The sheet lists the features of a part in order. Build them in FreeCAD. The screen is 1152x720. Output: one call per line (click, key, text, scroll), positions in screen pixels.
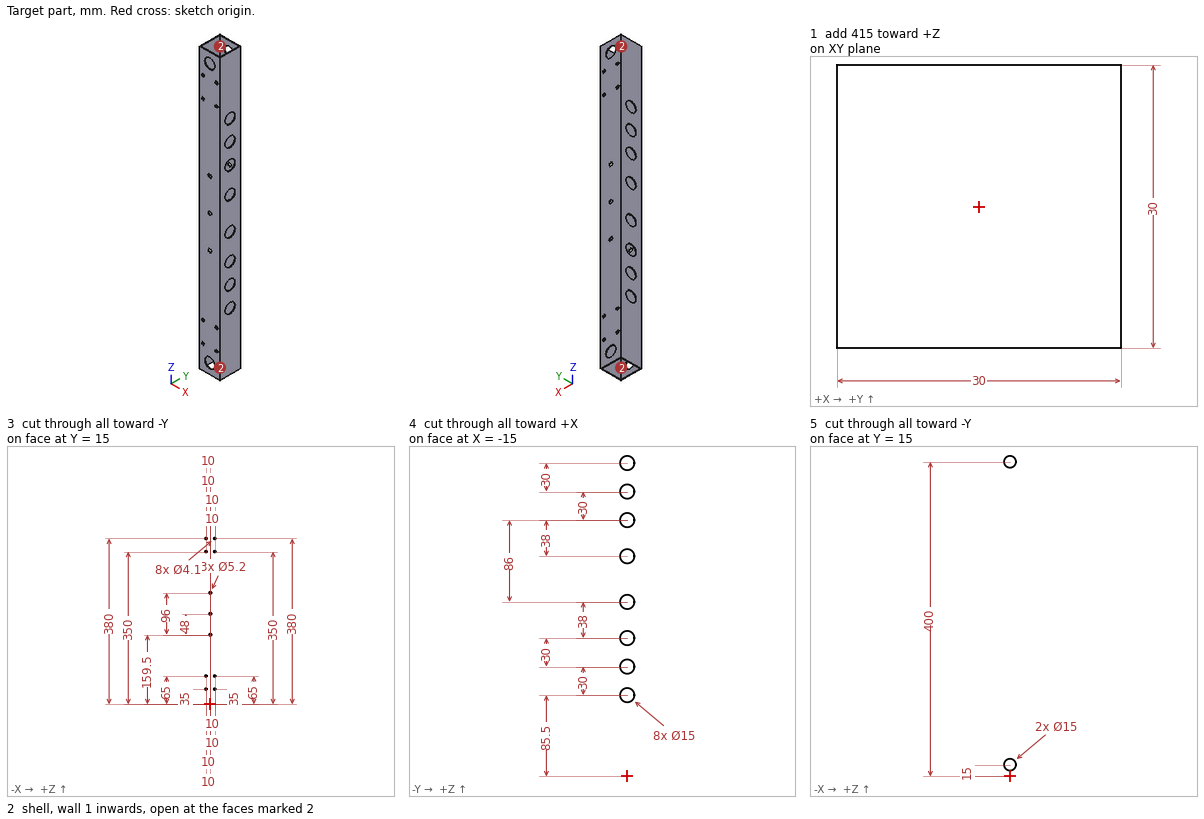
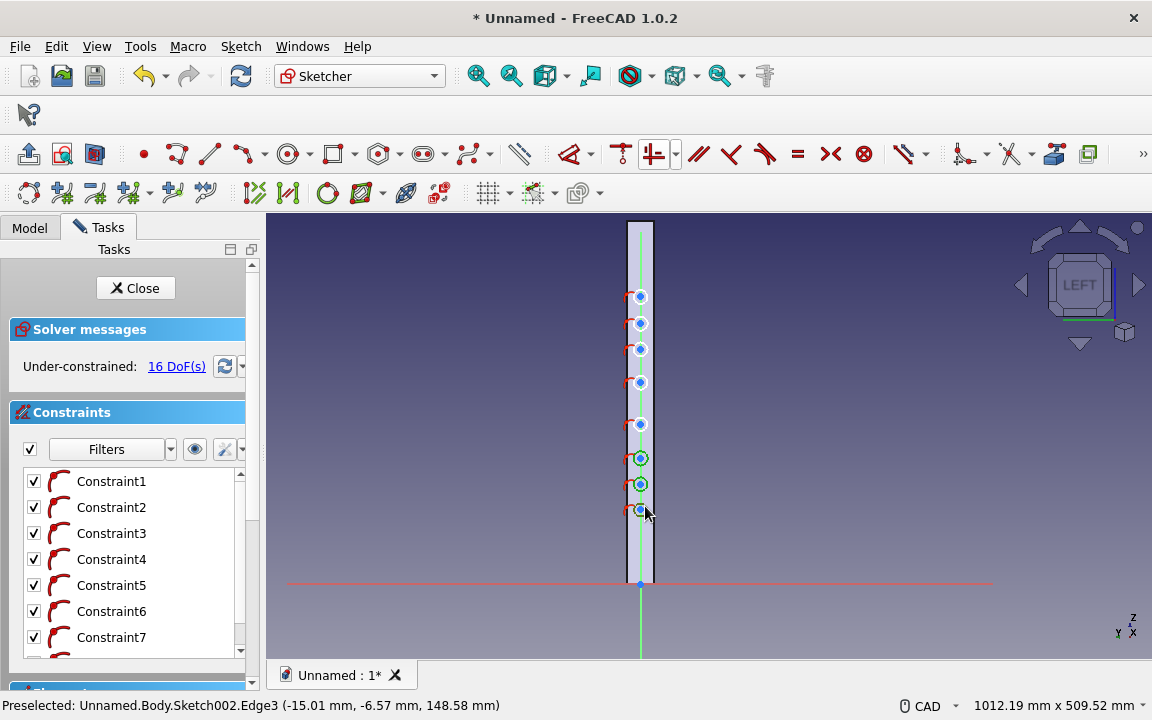
scroll(645, 345, up, 6)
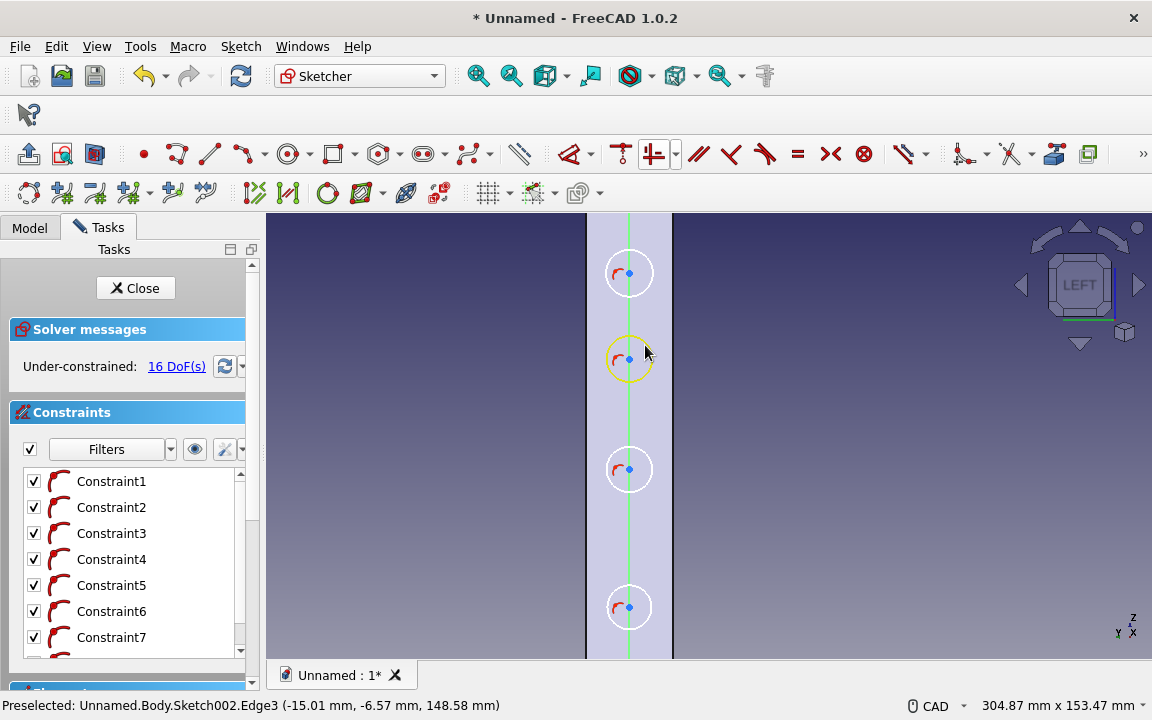
click(646, 343)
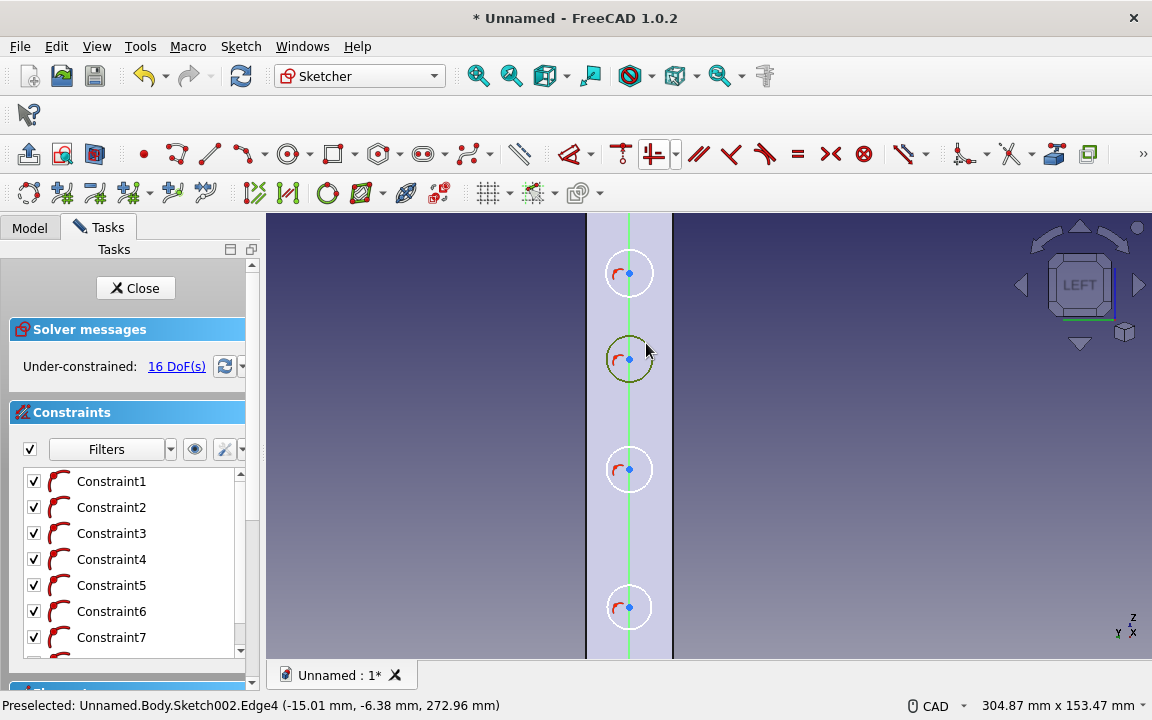
click(646, 257)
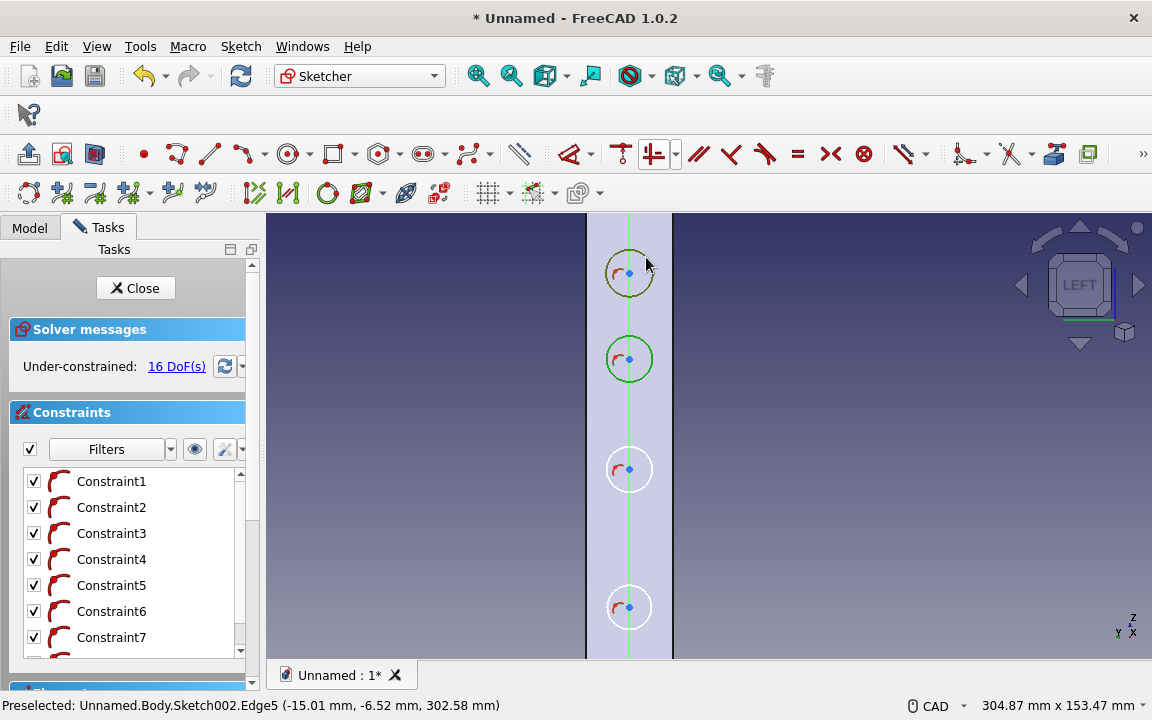
scroll(645, 344, down, 6)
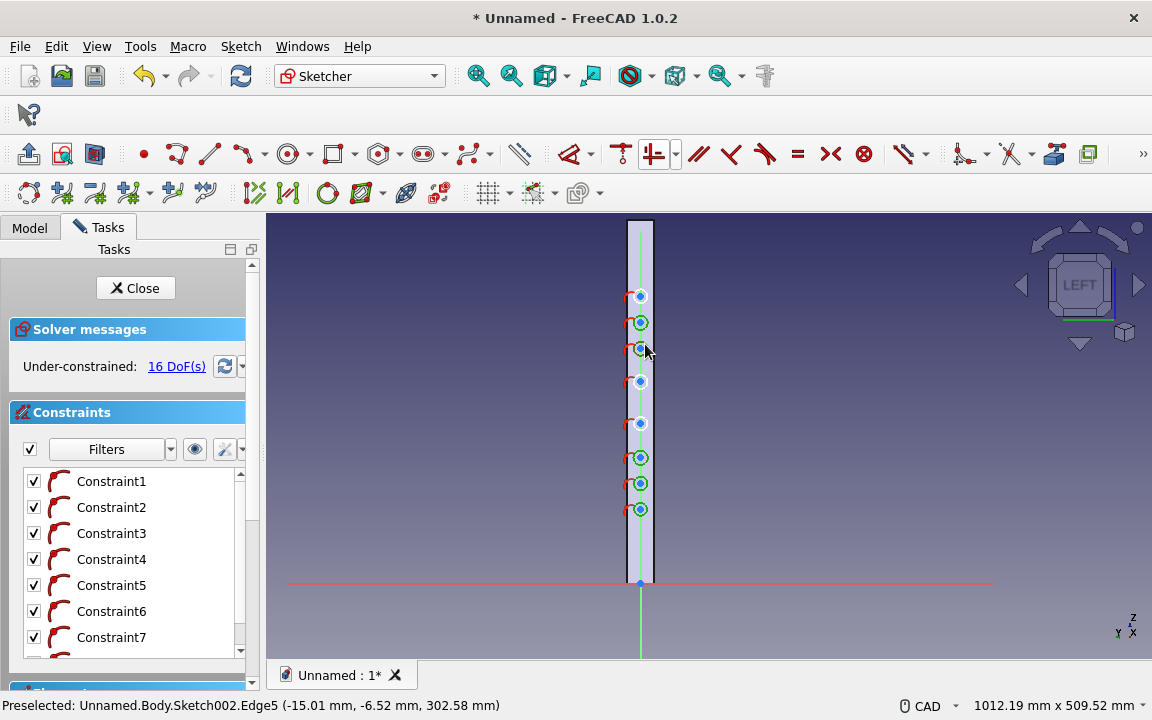
scroll(645, 291, up, 6)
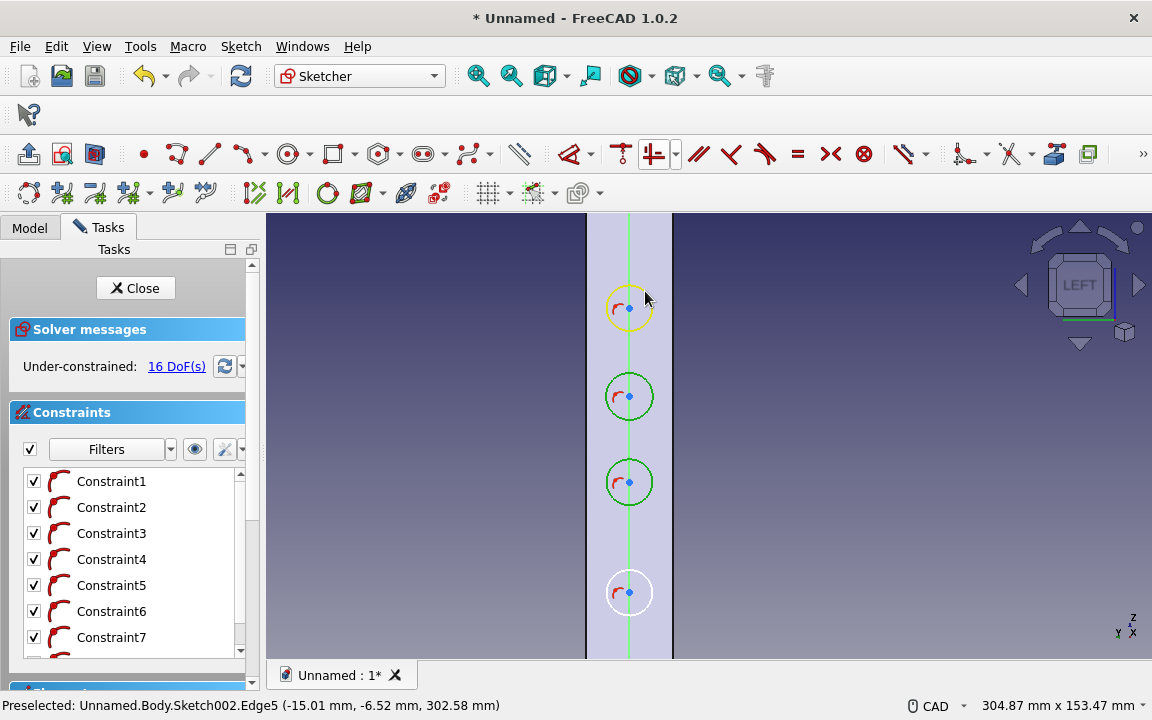
click(645, 292)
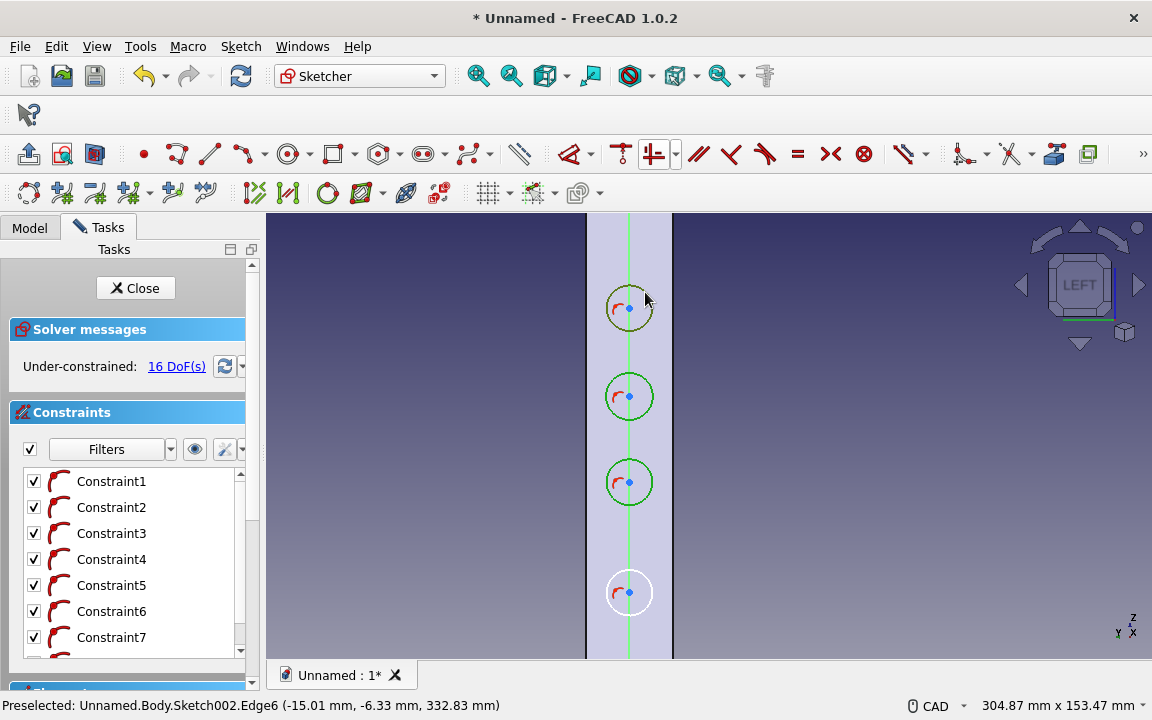
scroll(645, 291, down, 6)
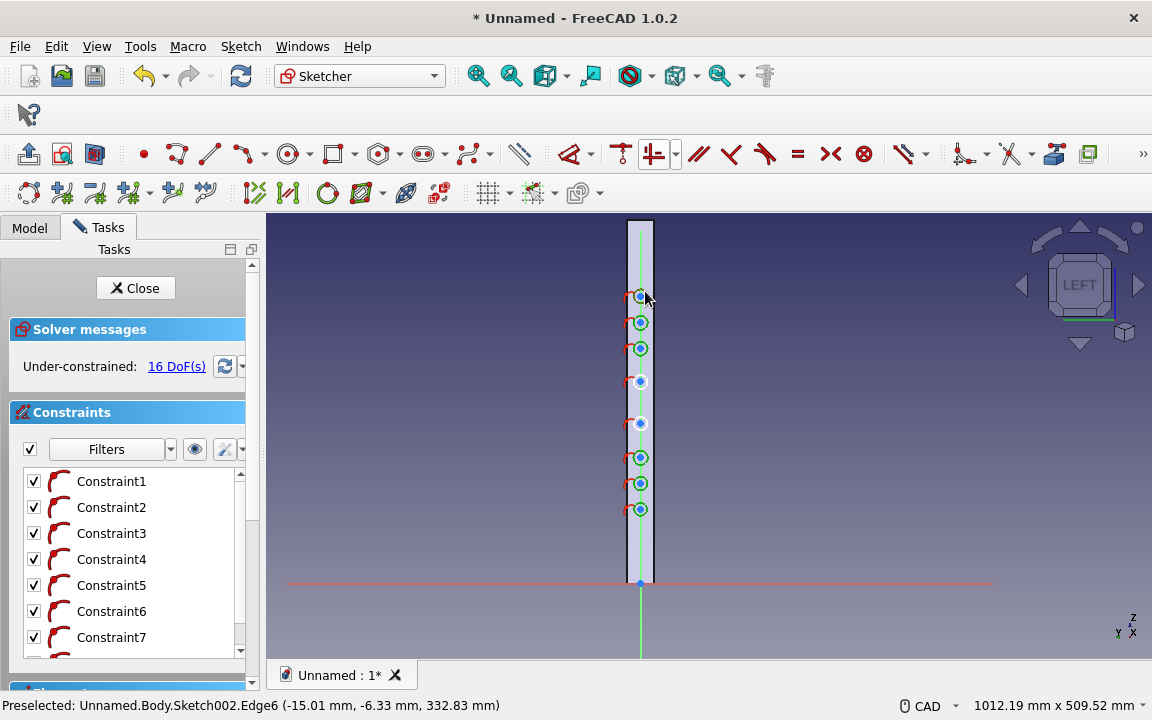
scroll(645, 419, up, 6)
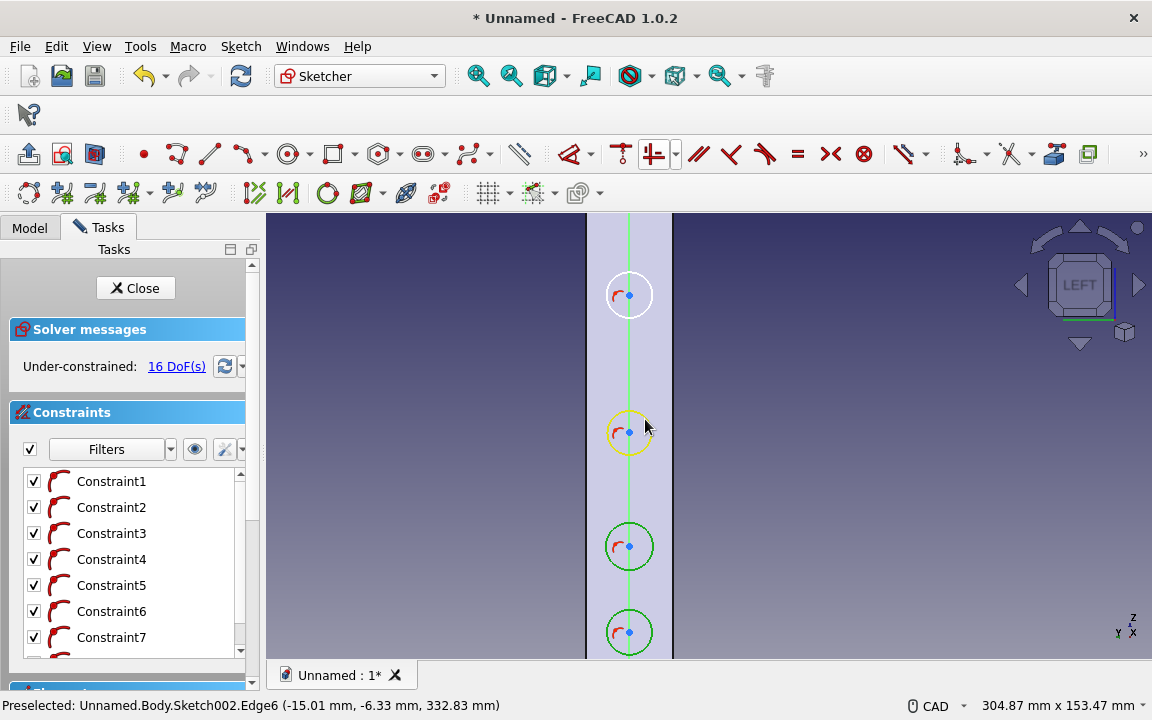
click(645, 417)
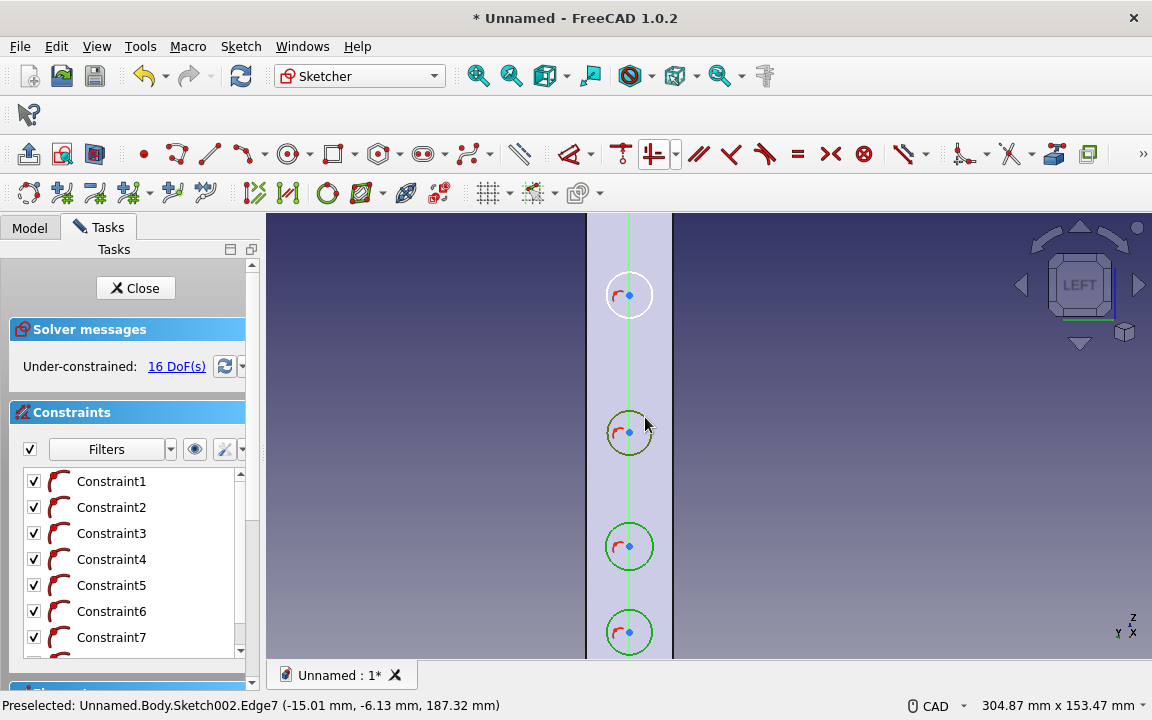
click(646, 279)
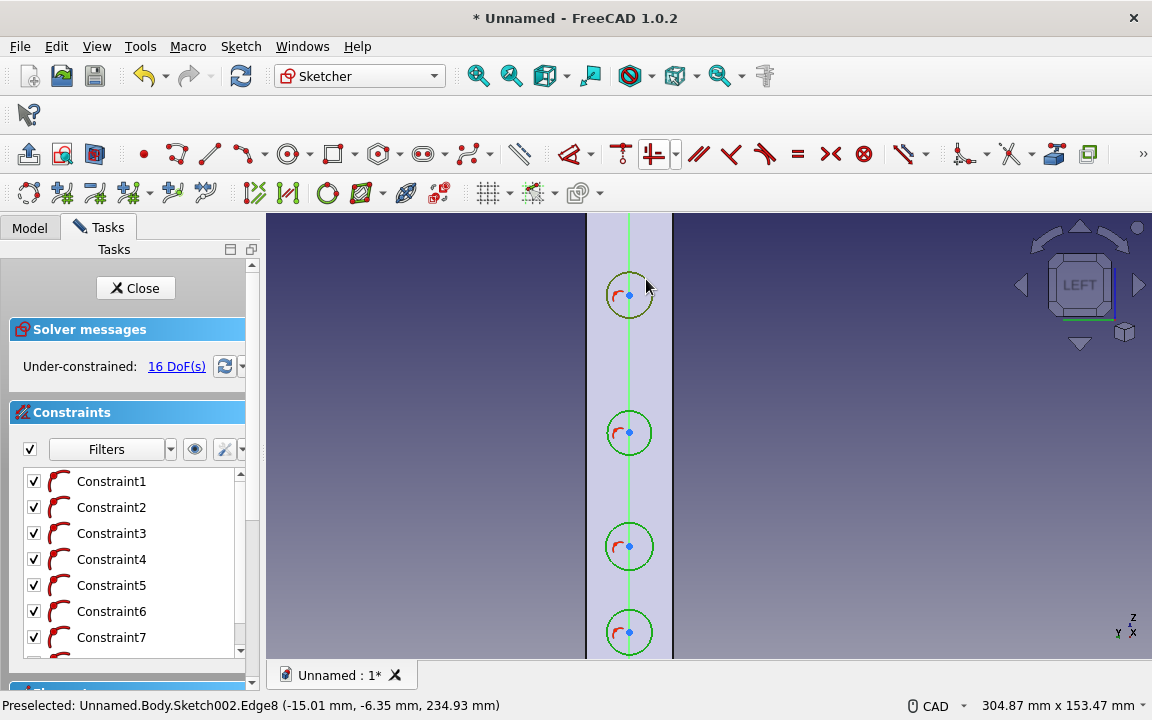
click(798, 154)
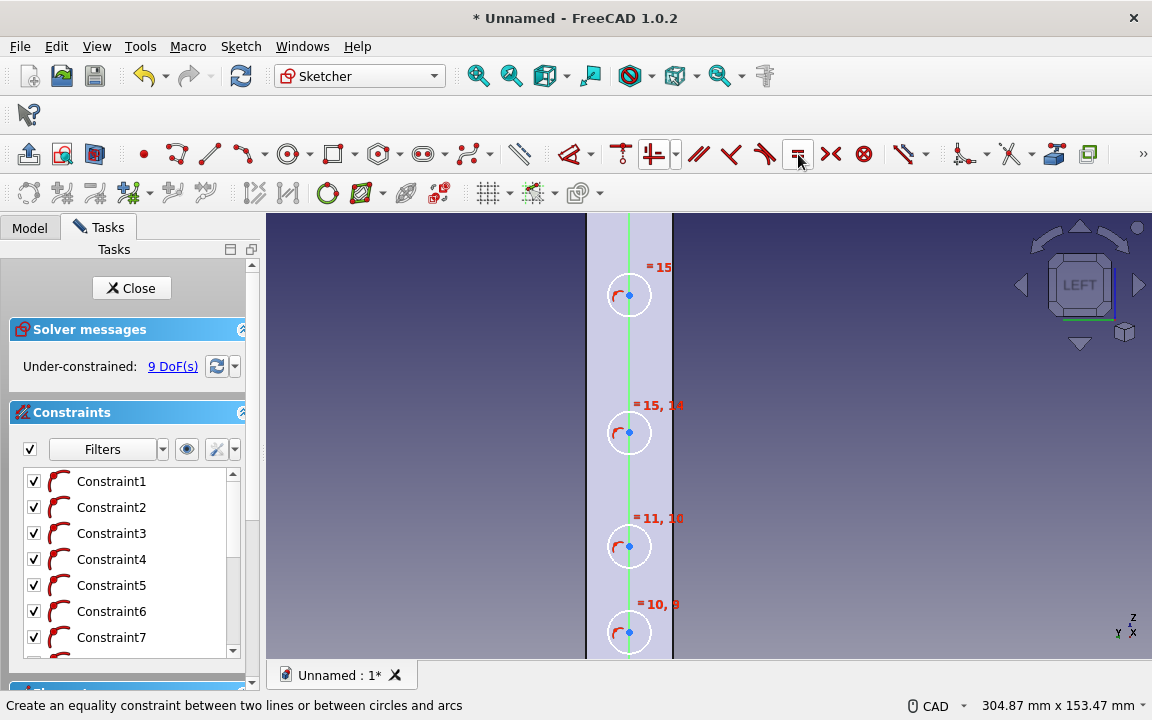
key(d)